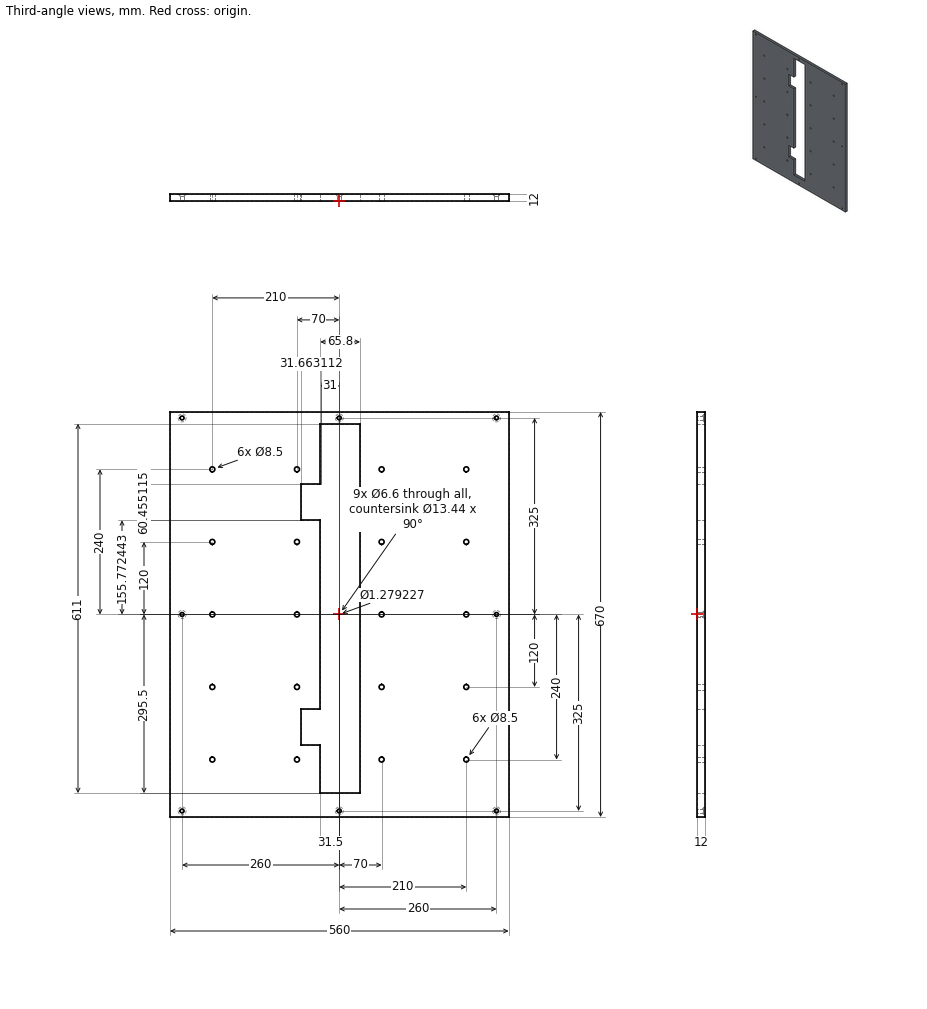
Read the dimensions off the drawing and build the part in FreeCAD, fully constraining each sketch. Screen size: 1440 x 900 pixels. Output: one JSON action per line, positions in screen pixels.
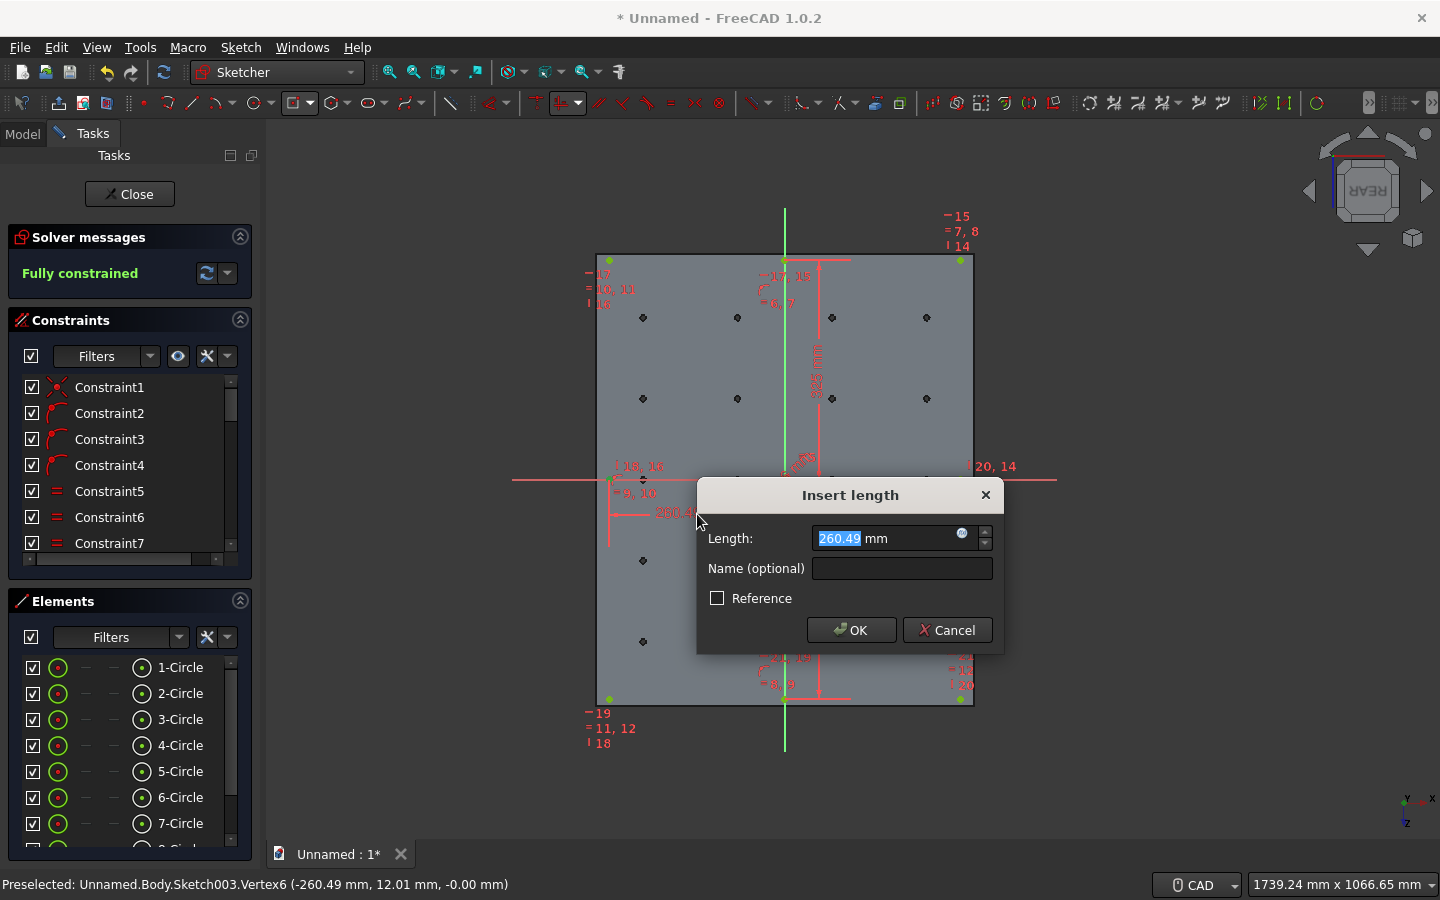
{"action": "type", "text": "260"}
{"action": "key", "text": "Return"}
{"action": "key", "text": "Escape"}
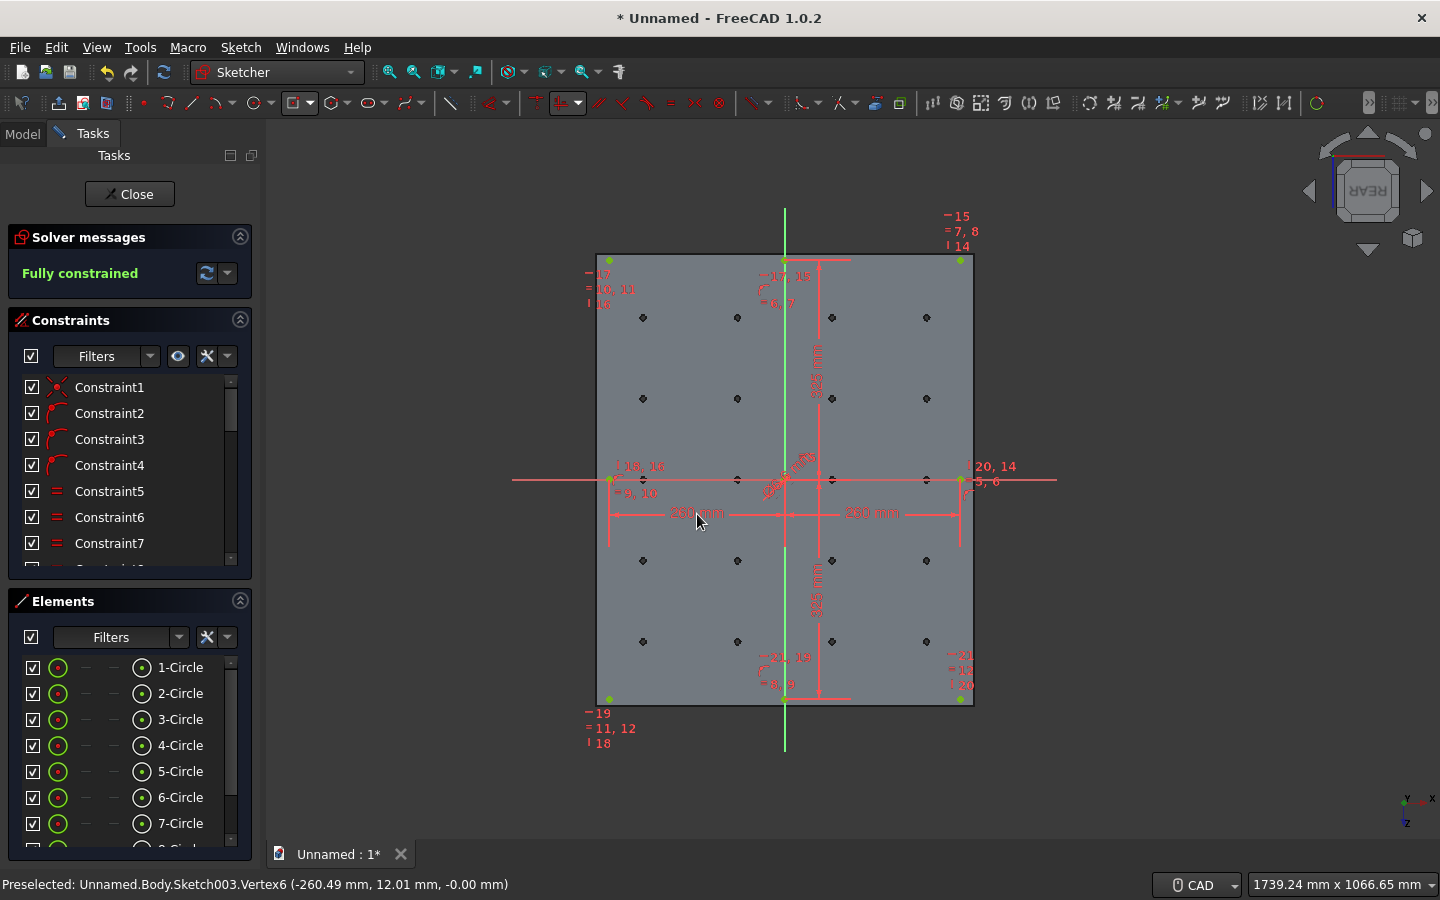
{"action": "left_click", "coordinate": [130, 194]}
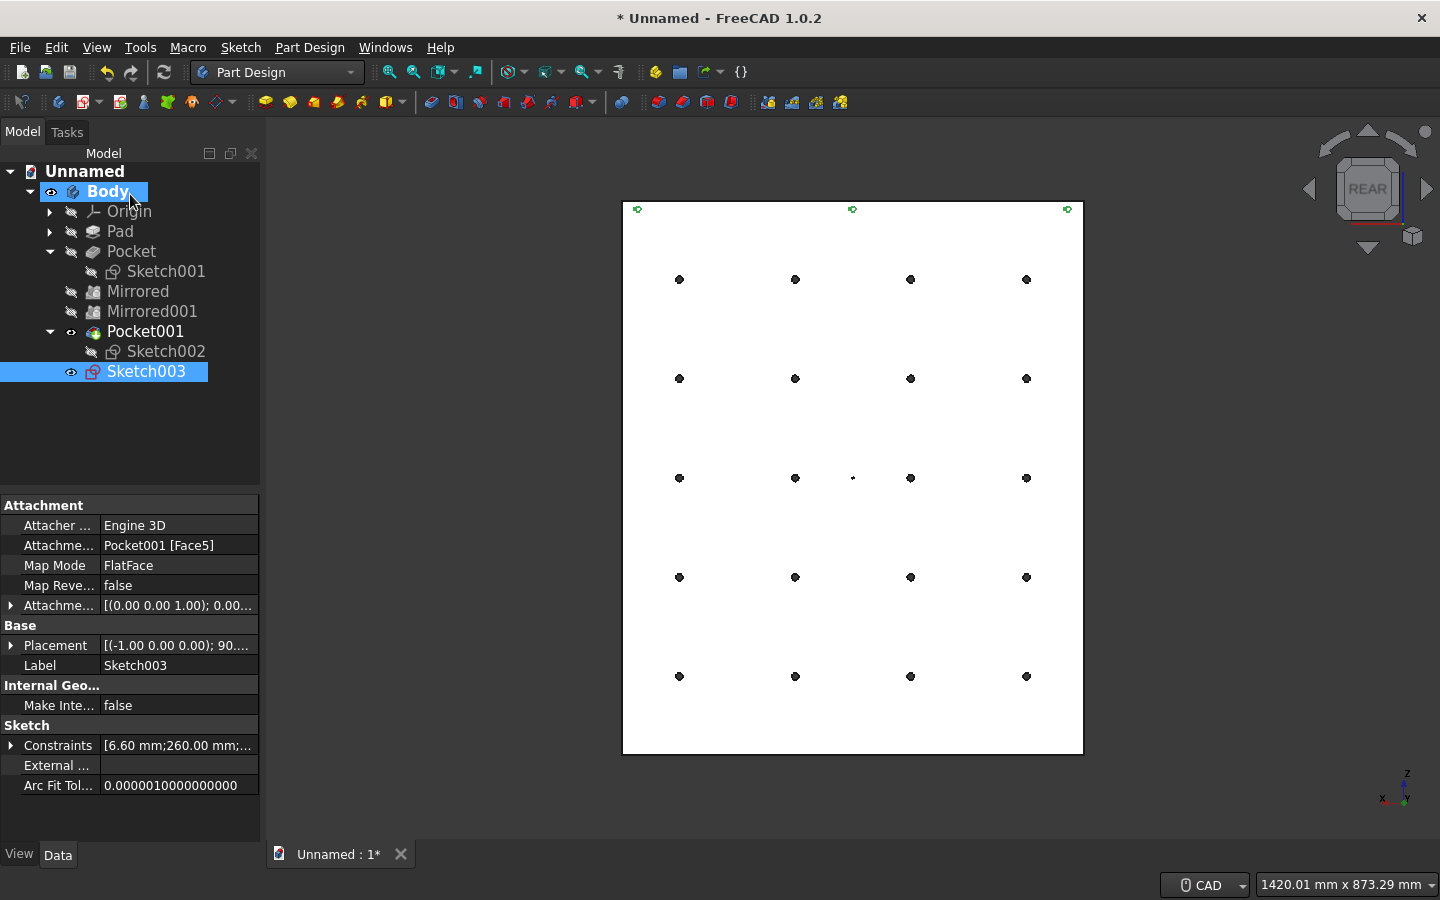
{"action": "left_click", "coordinate": [456, 102]}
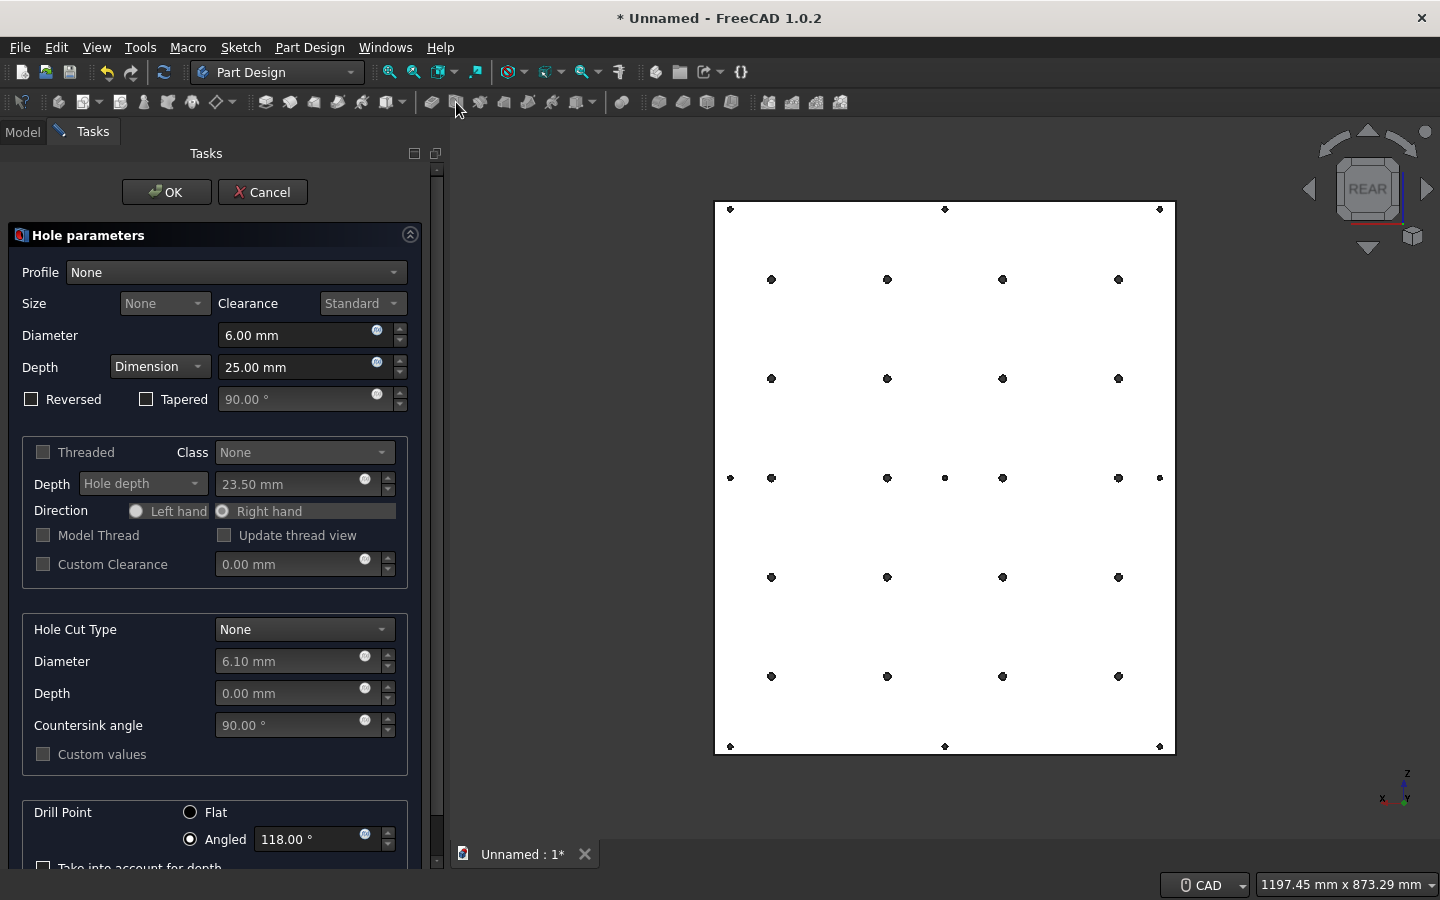
{"action": "triple_click", "coordinate": [305, 335]}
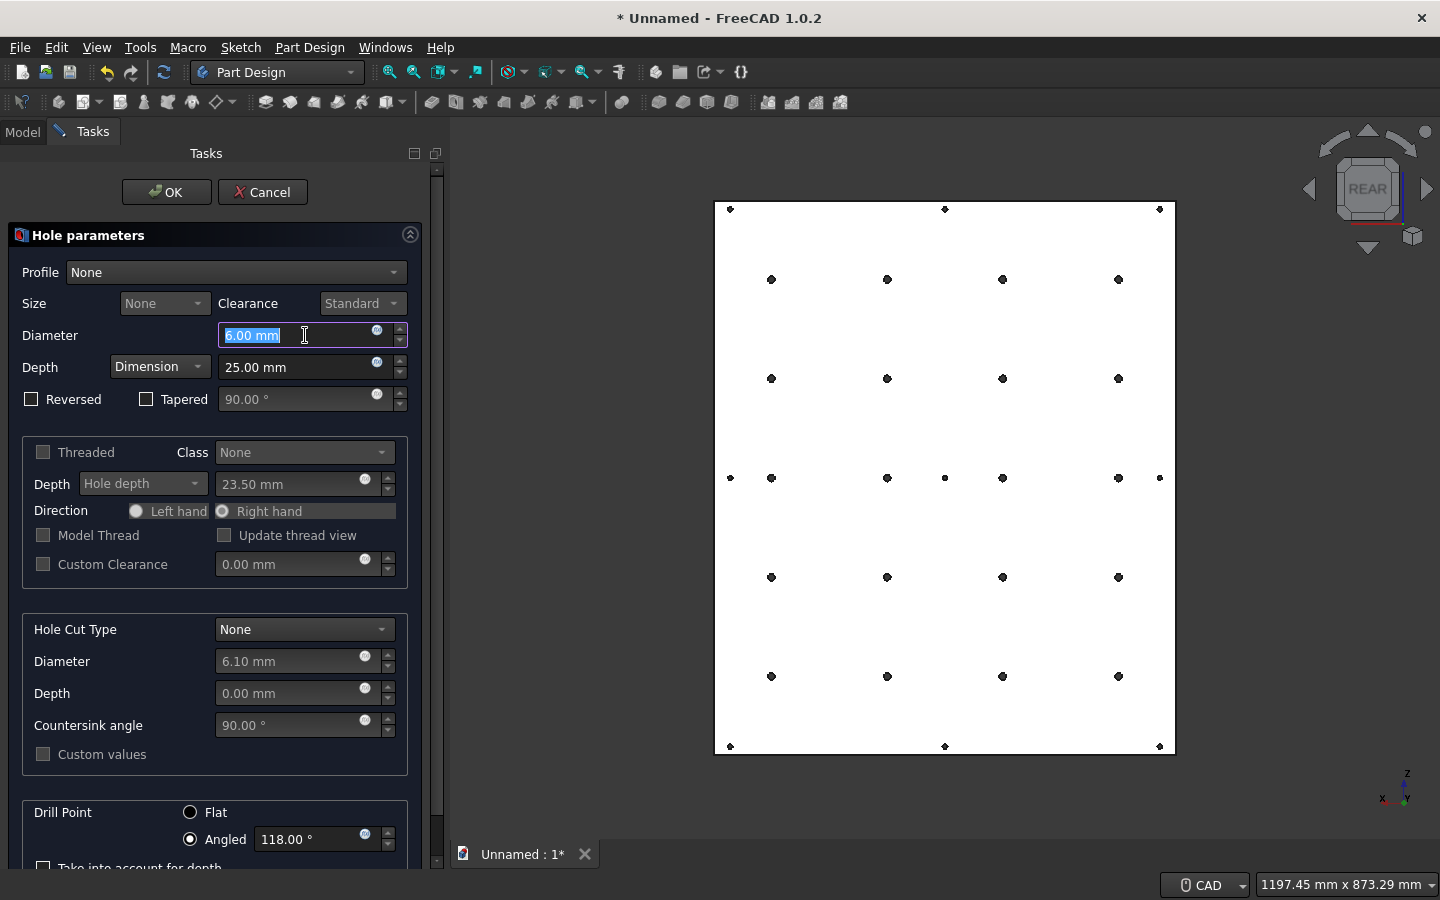
{"action": "type", "text": "6.6"}
{"action": "key", "text": "Tab"}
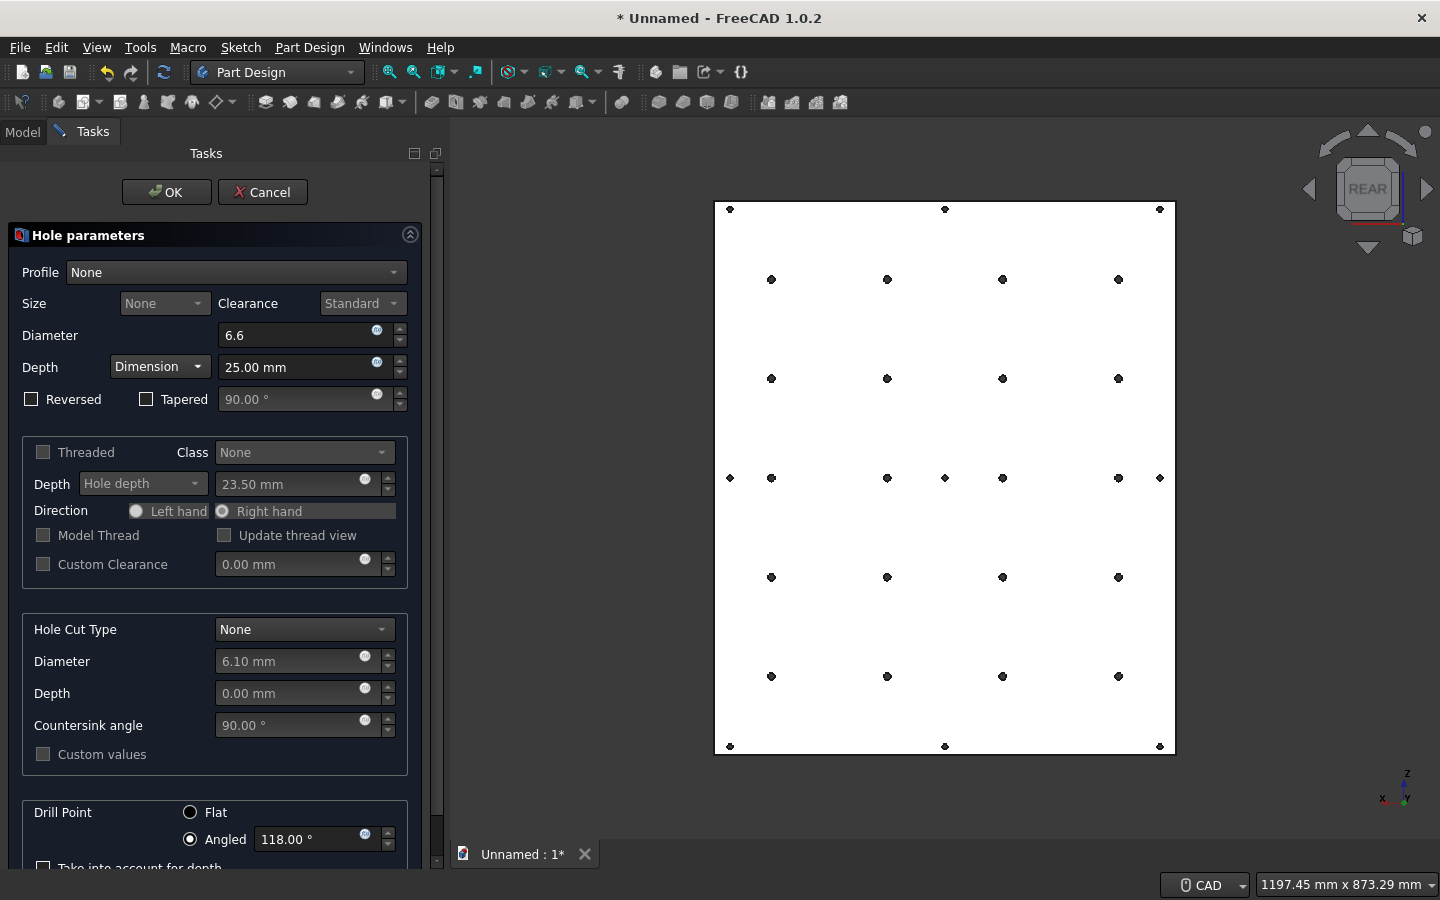
{"action": "left_click", "coordinate": [161, 366]}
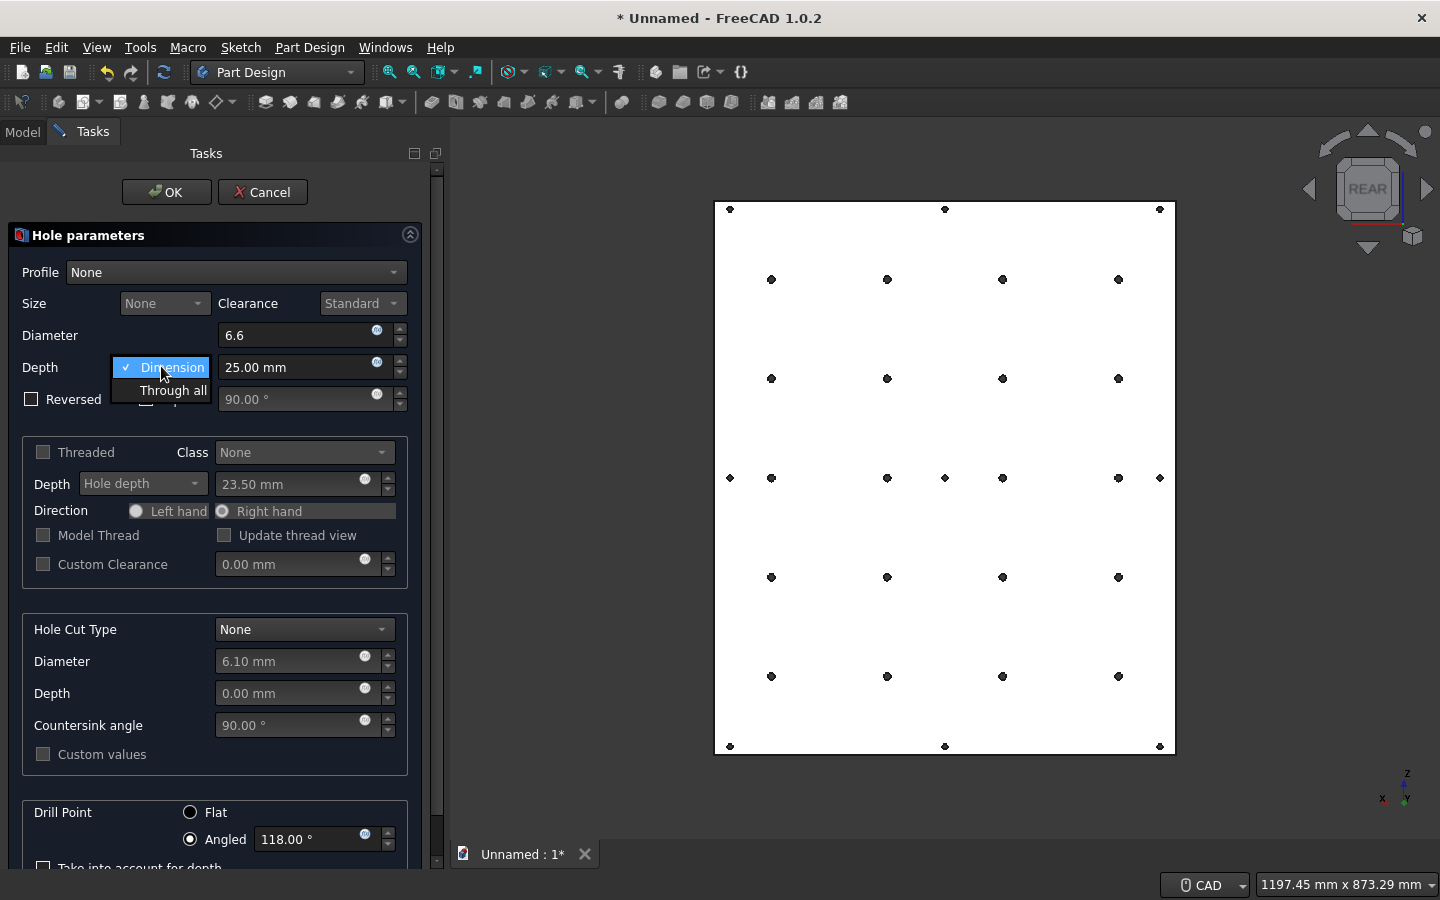
{"action": "left_click", "coordinate": [160, 390]}